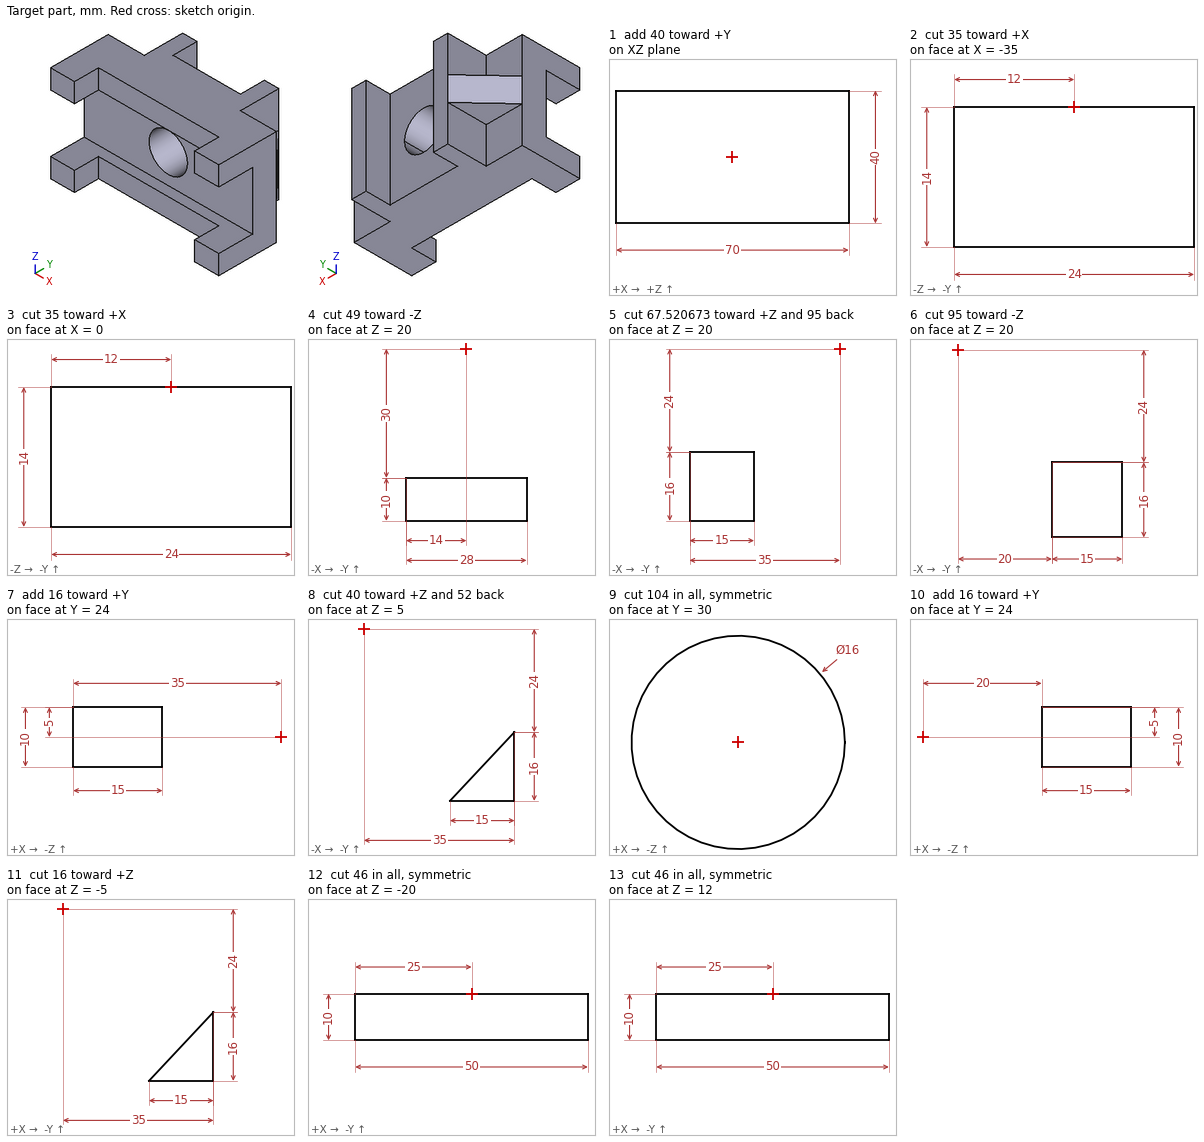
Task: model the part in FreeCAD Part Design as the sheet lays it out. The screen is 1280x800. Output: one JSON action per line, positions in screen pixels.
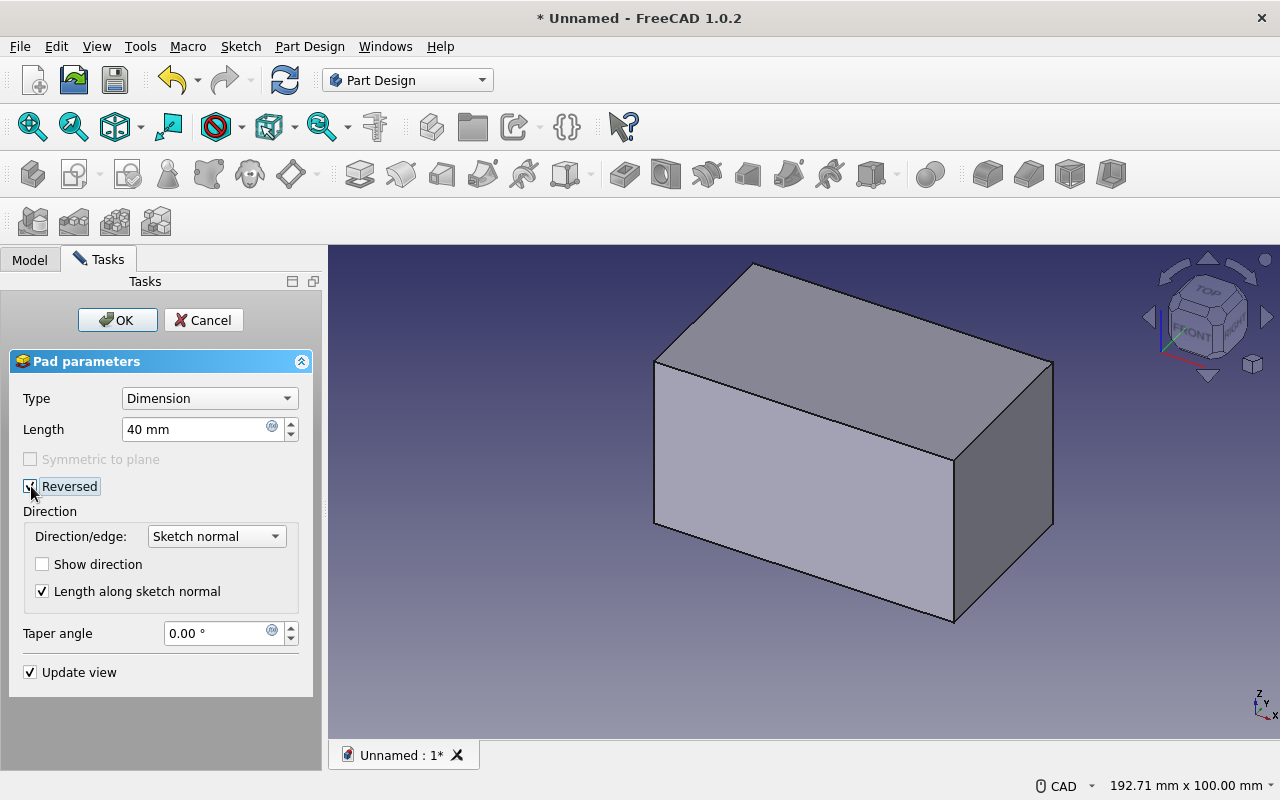
{"action": "left_click", "coordinate": [118, 320]}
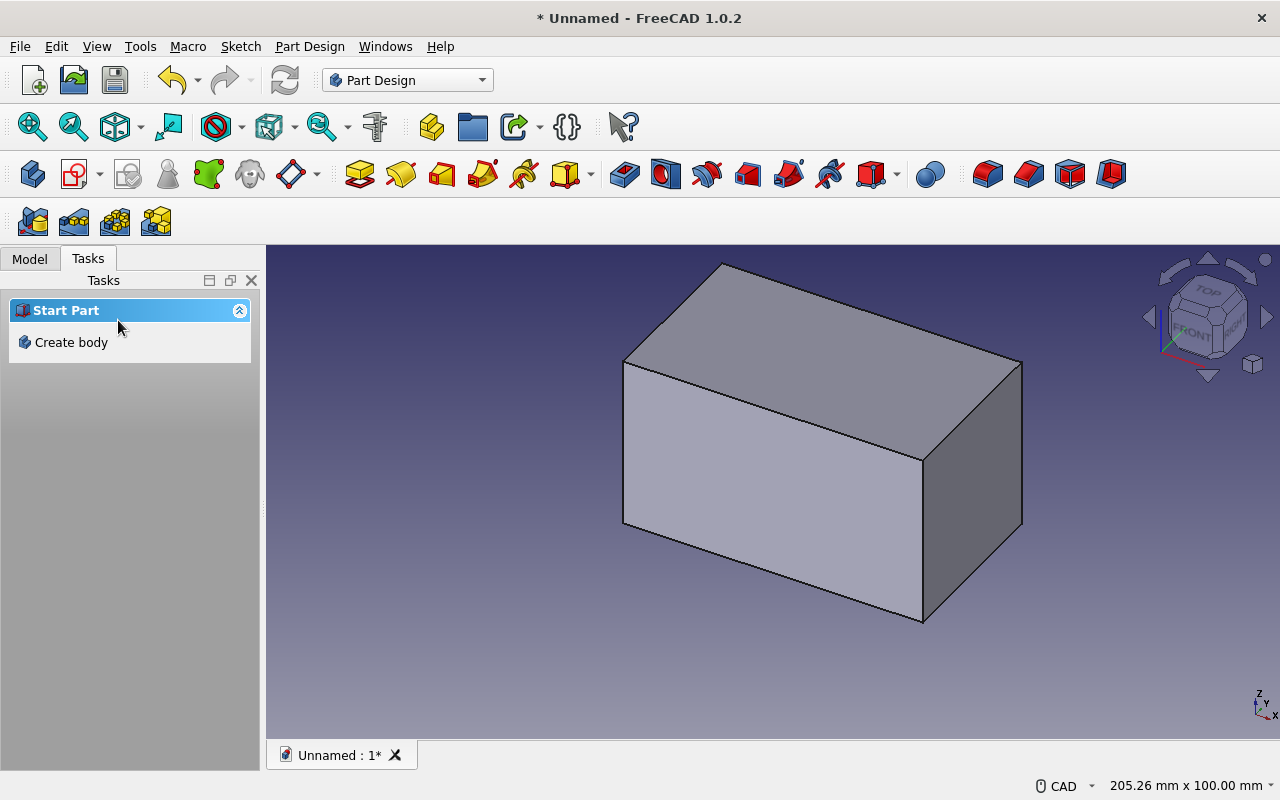
{"action": "key", "text": "6"}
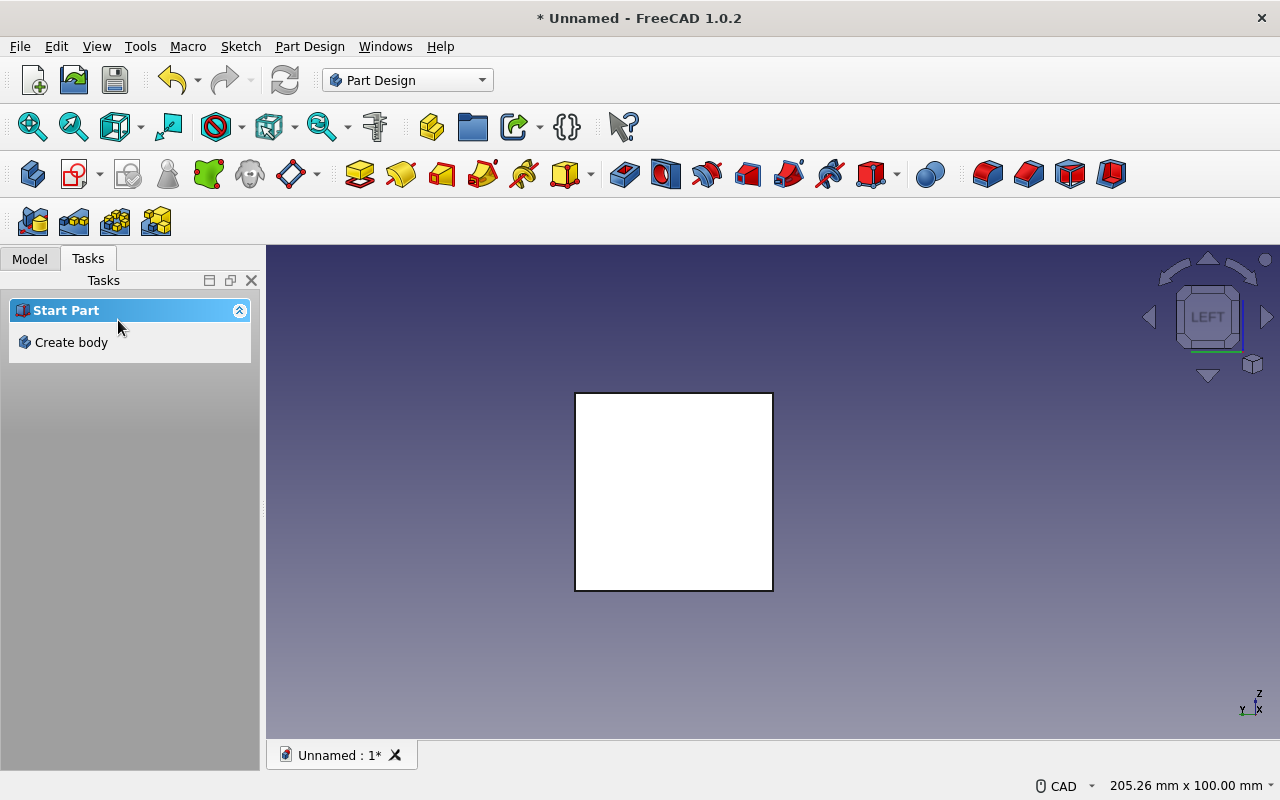
{"action": "left_click", "coordinate": [33, 128]}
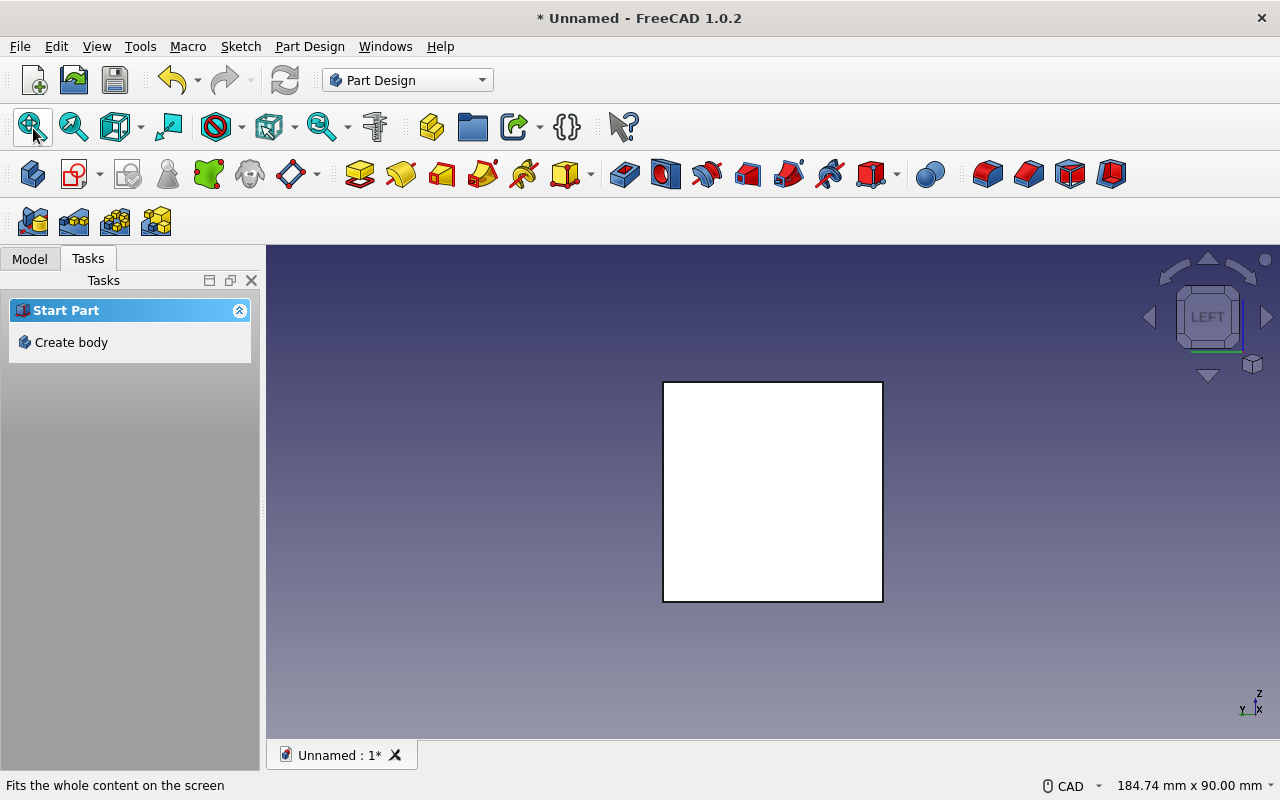
{"action": "left_click", "coordinate": [773, 491]}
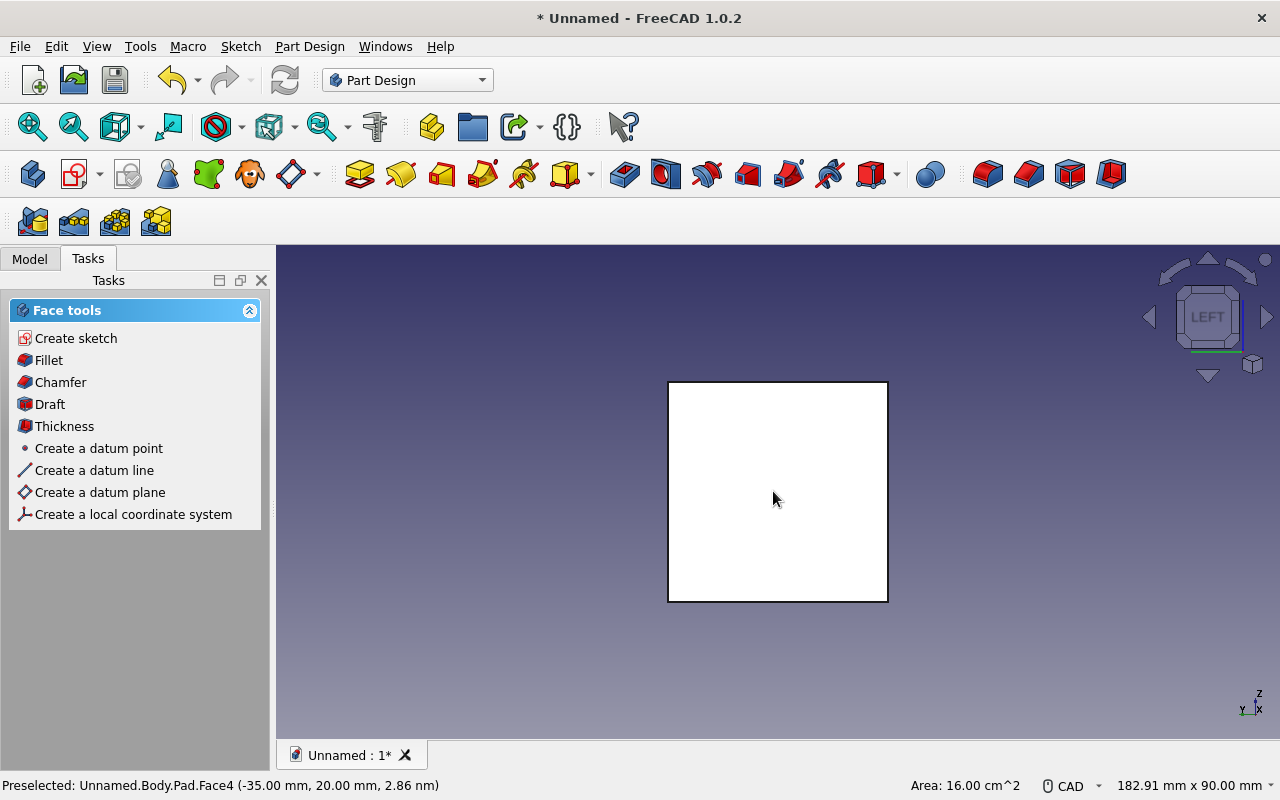
{"action": "left_click", "coordinate": [74, 174]}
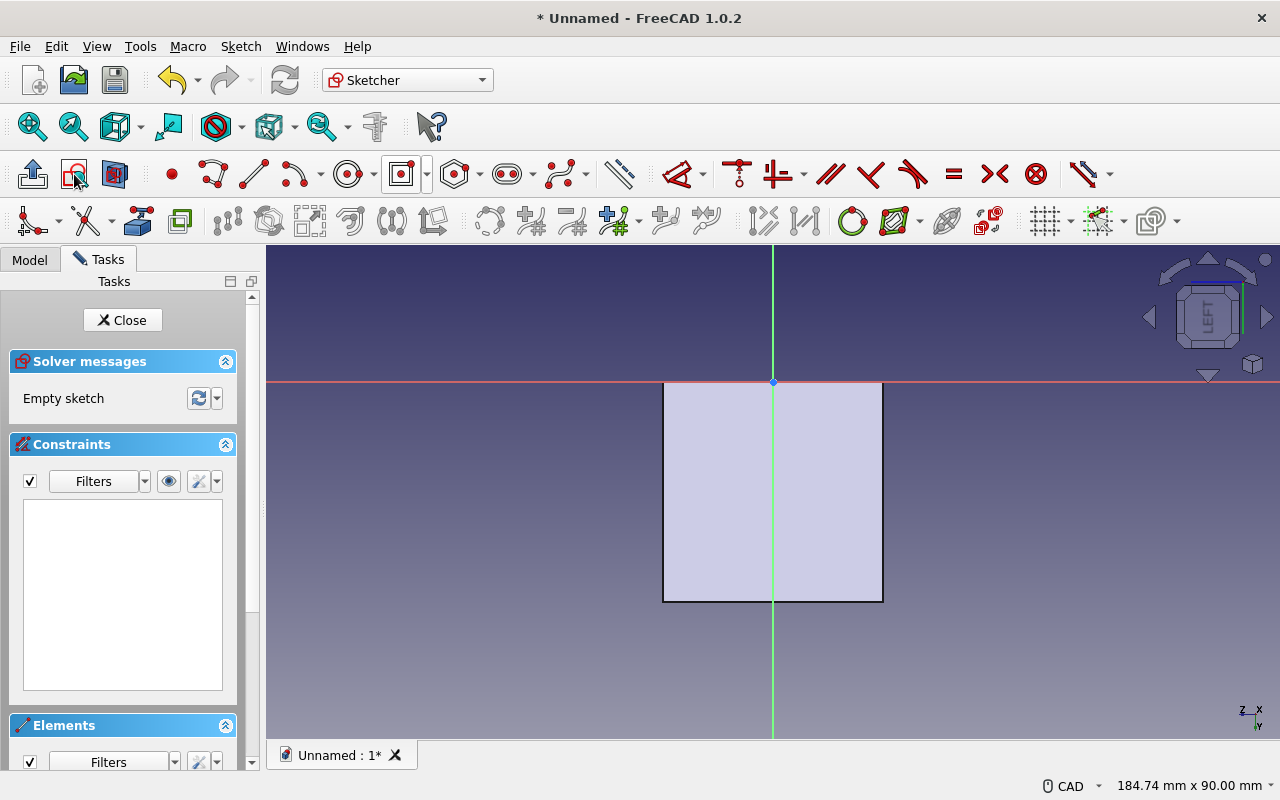
{"action": "scroll", "coordinate": [795, 397], "scroll_direction": "up", "scroll_amount": 7}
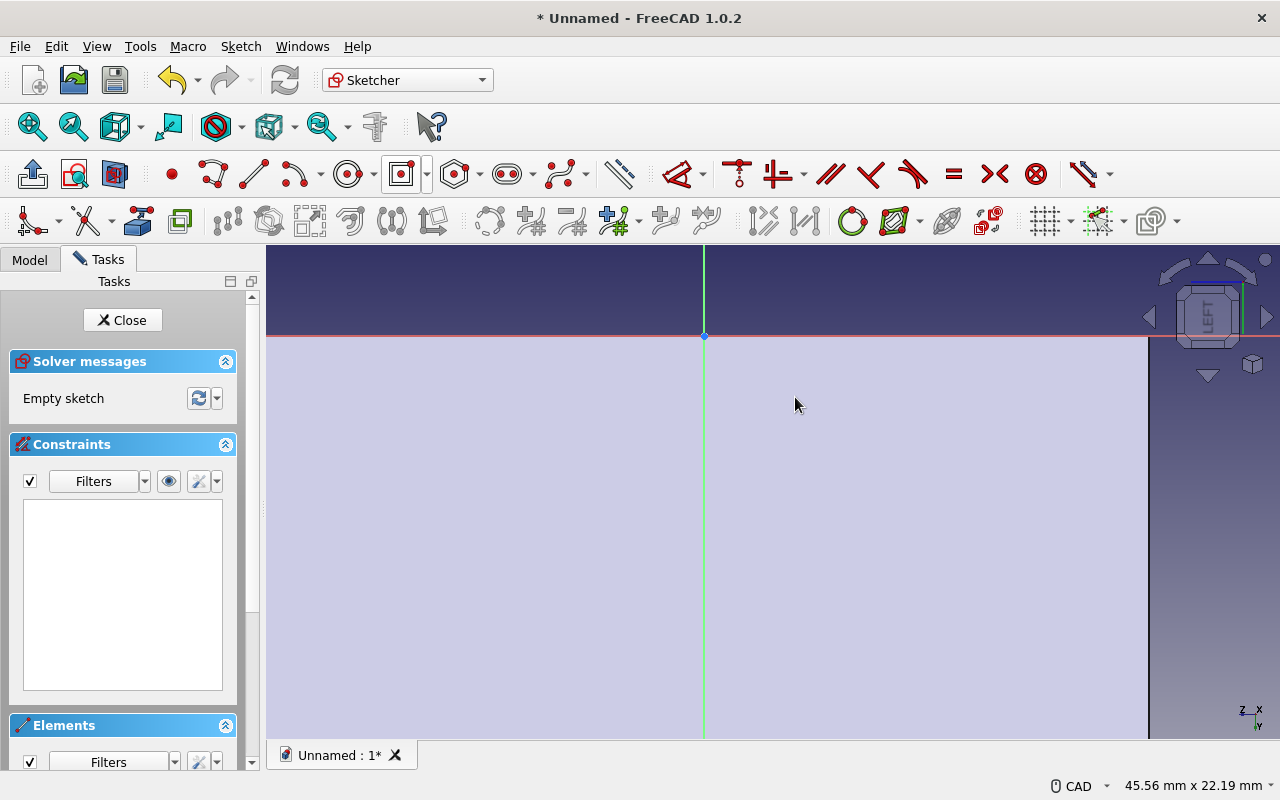
{"action": "key", "text": "g r"}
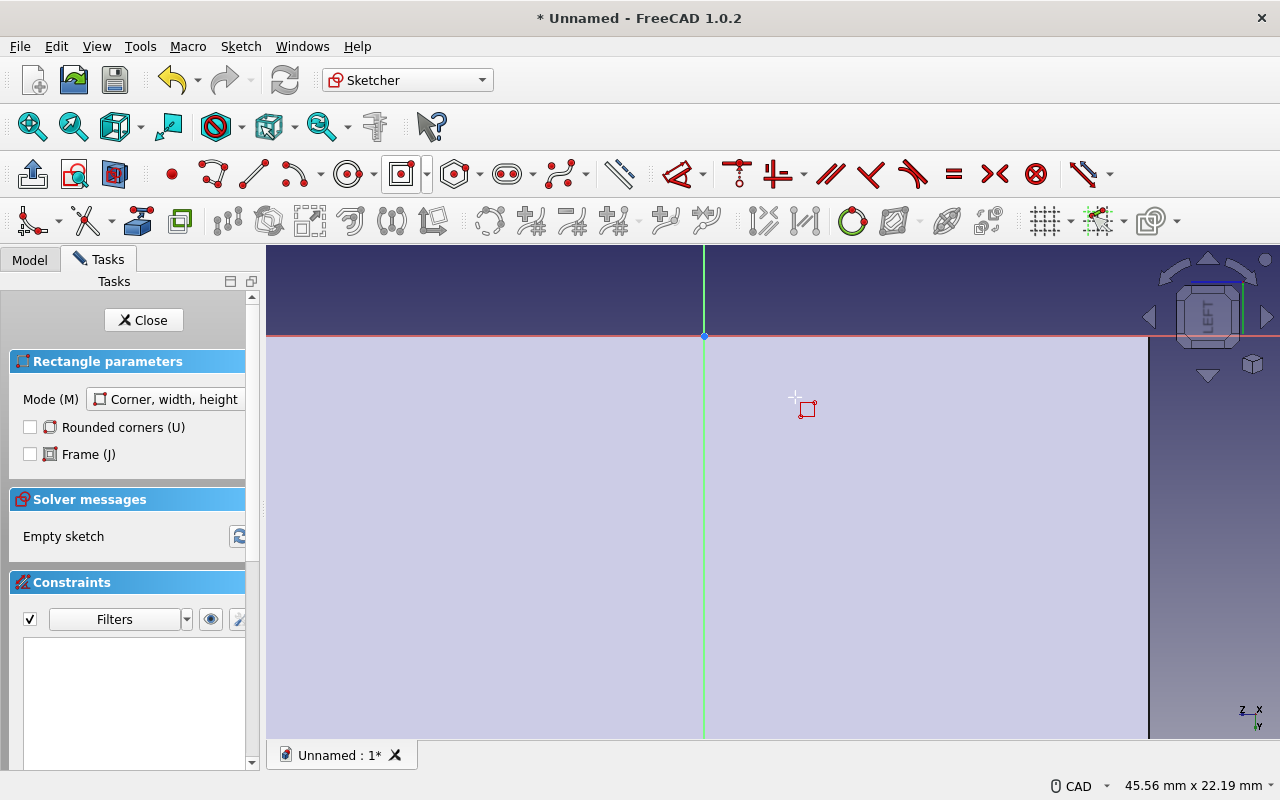
{"action": "left_click", "coordinate": [437, 336]}
{"action": "left_click", "coordinate": [971, 648]}
{"action": "key", "text": "Escape"}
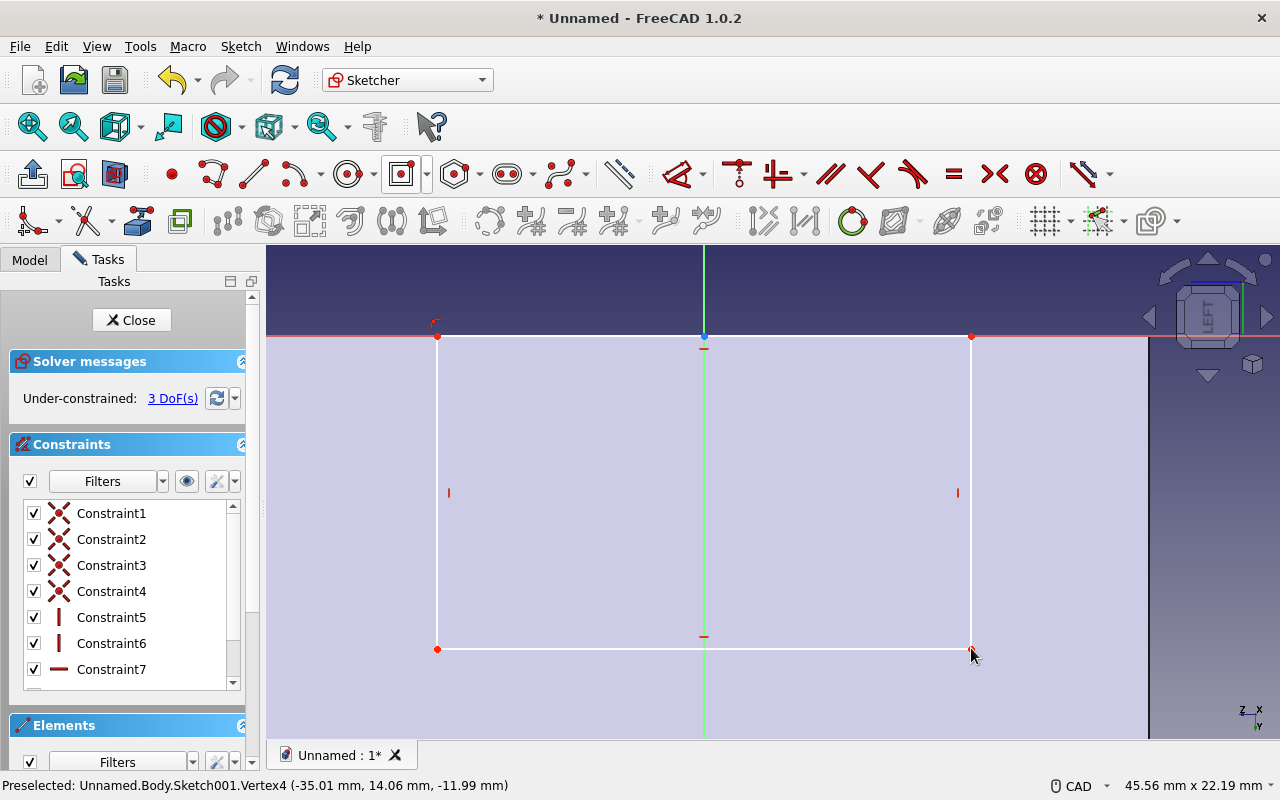
{"action": "left_click", "coordinate": [437, 430]}